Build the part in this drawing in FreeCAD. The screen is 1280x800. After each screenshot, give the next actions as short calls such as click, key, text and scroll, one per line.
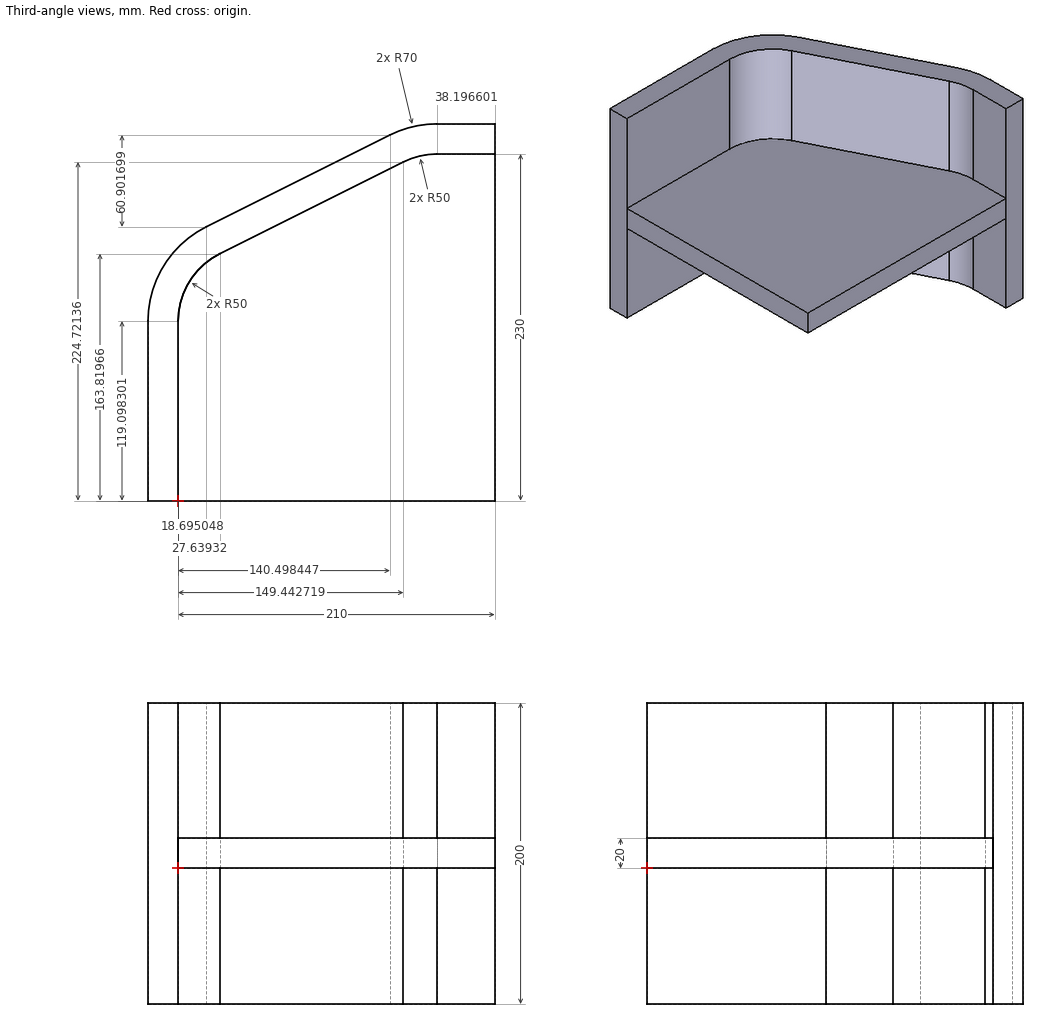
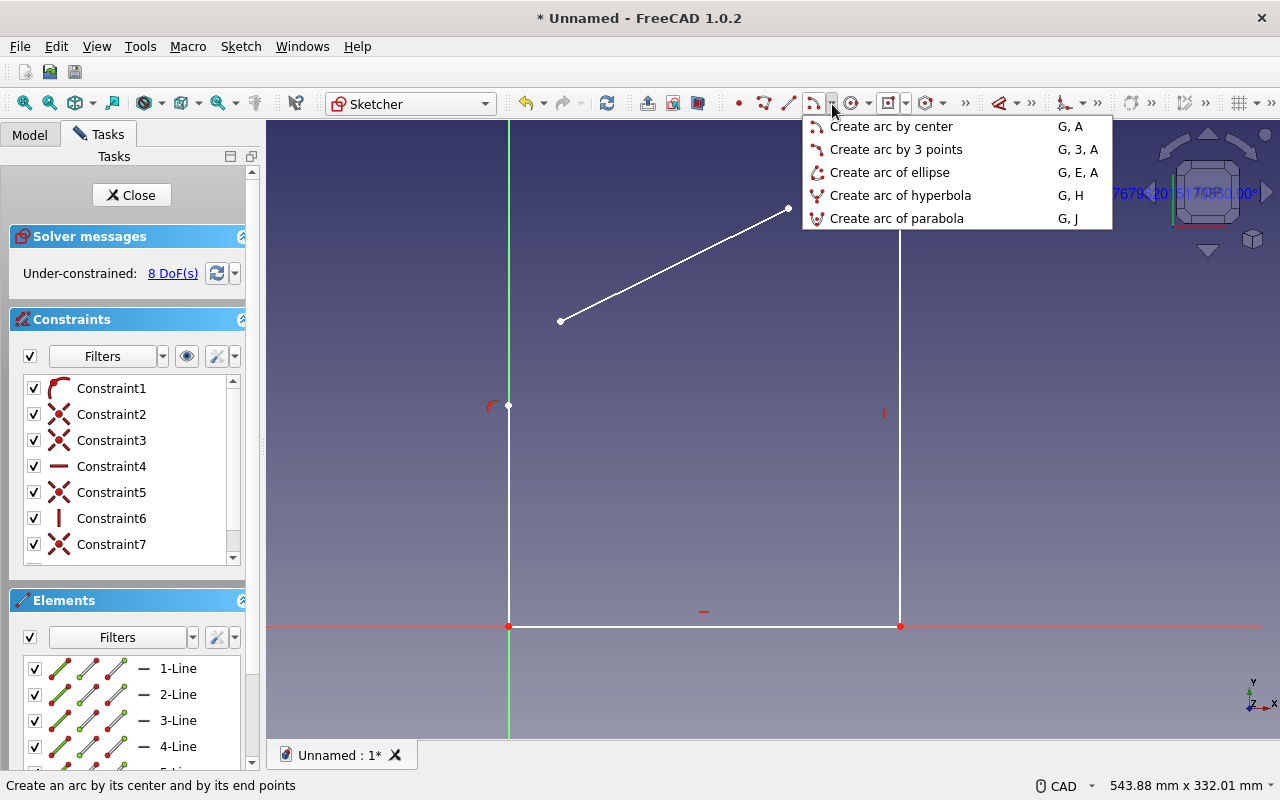
click(958, 150)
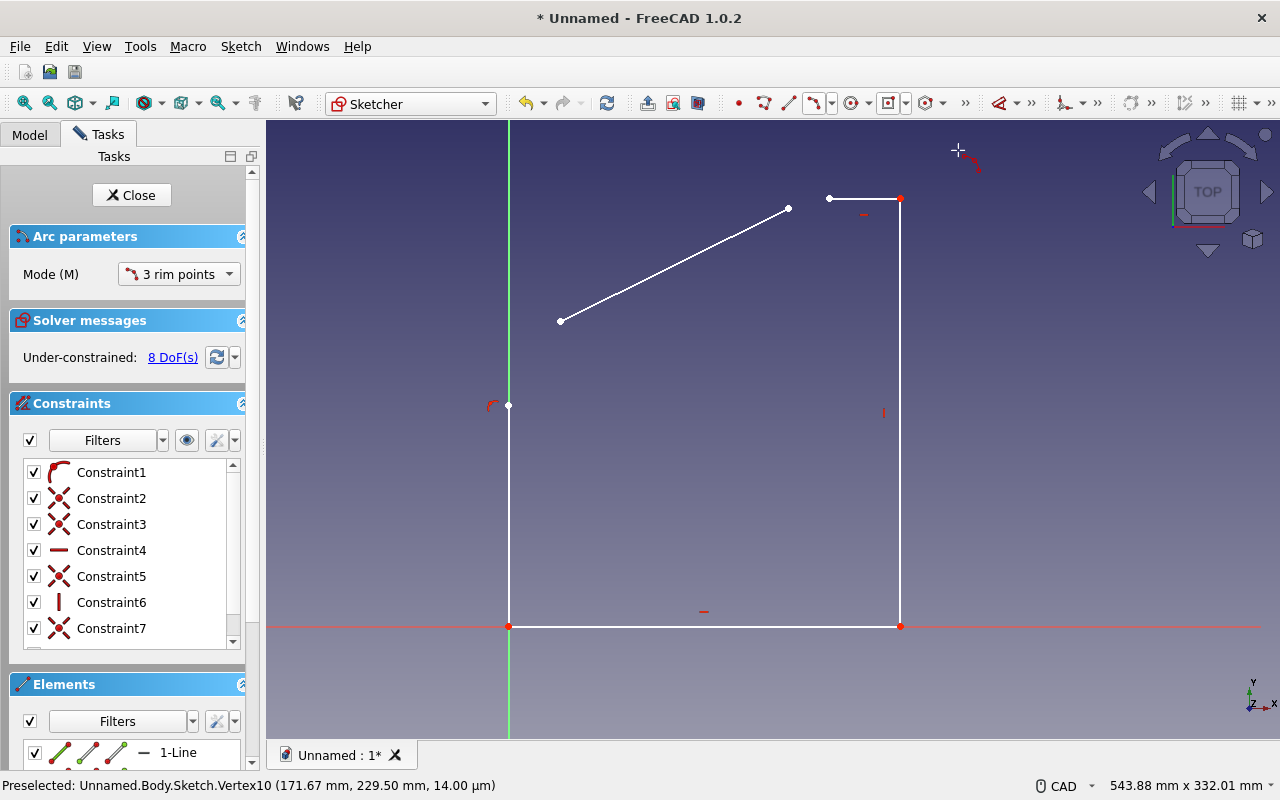
click(560, 322)
click(509, 406)
click(523, 356)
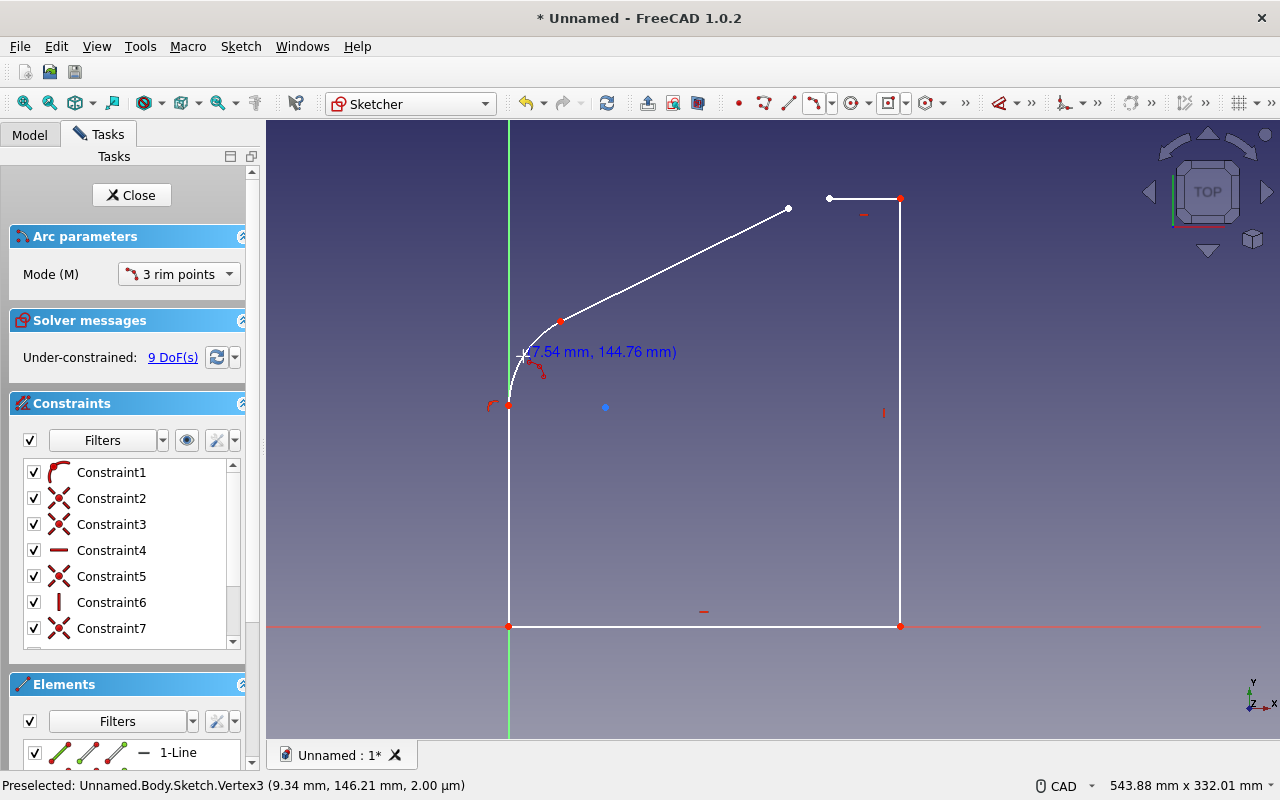
click(829, 199)
click(788, 209)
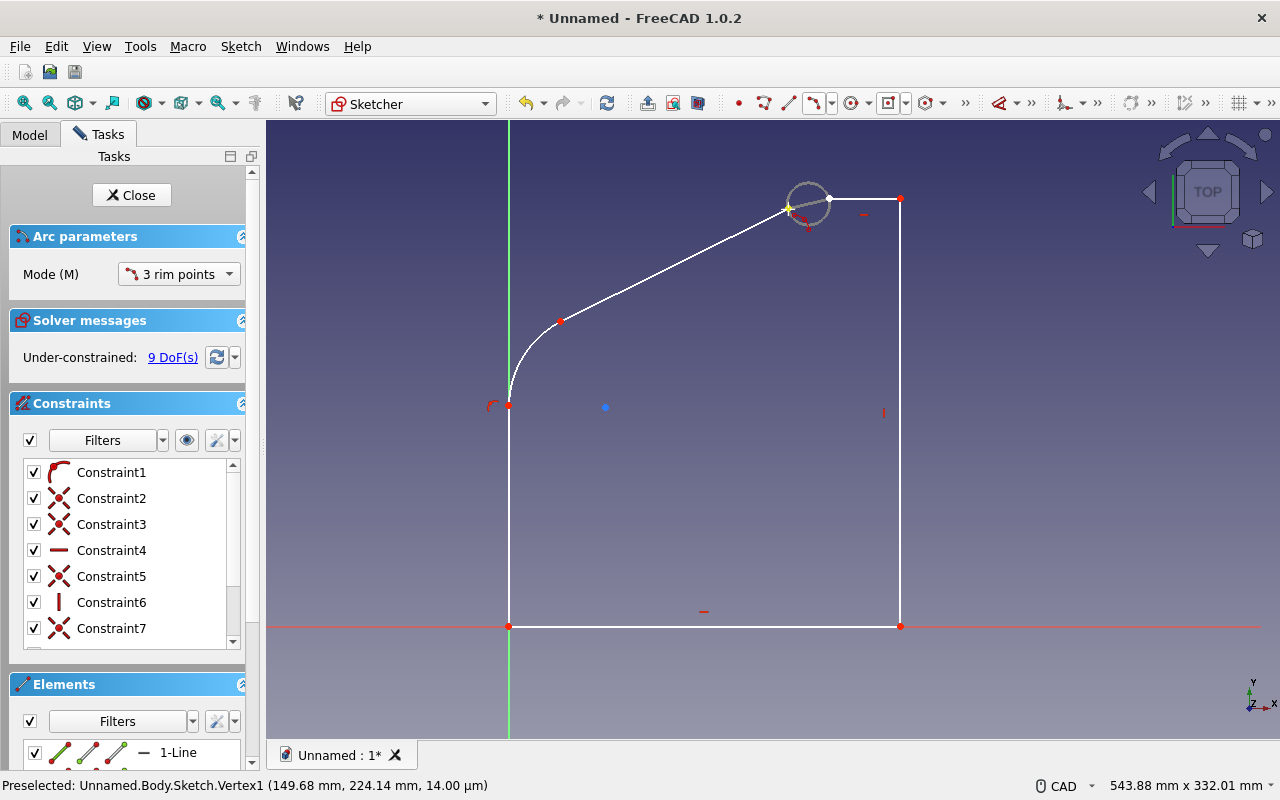
scroll(808, 201, up, 10)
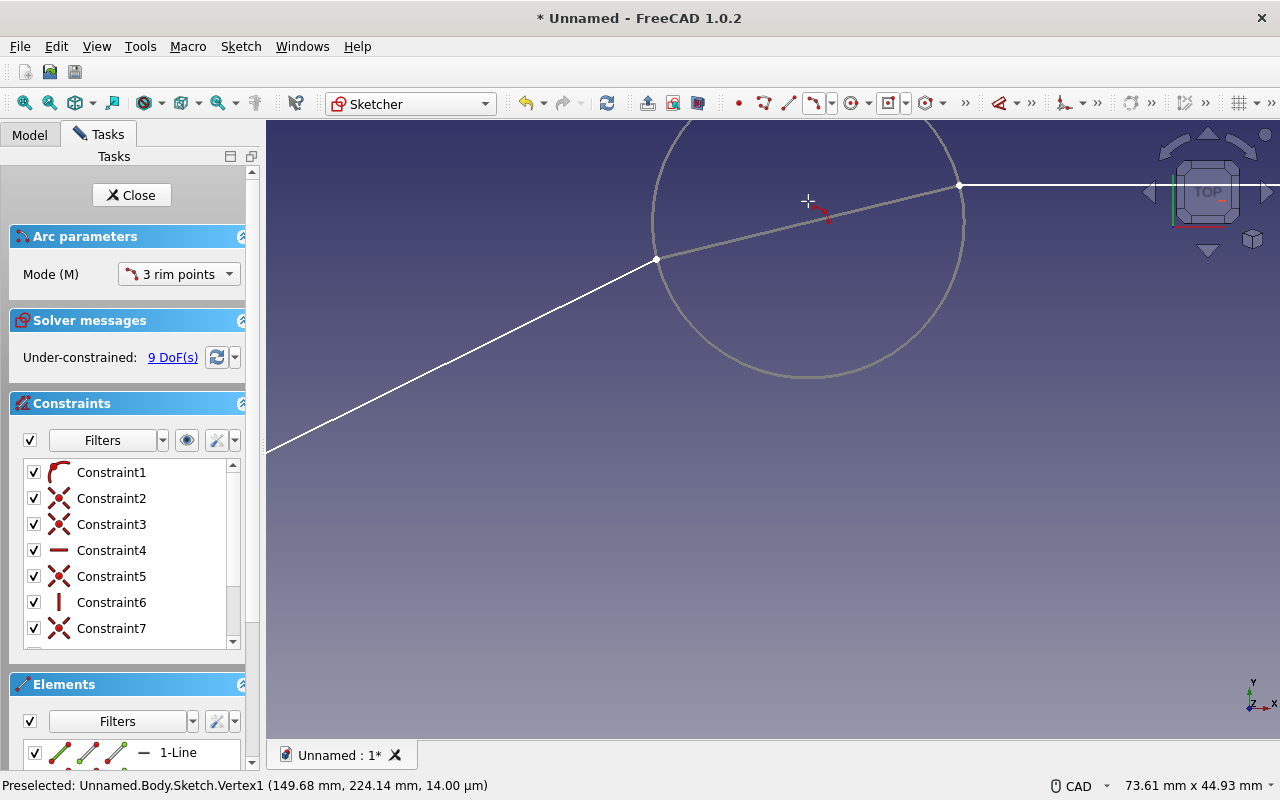
click(803, 197)
key(Escape)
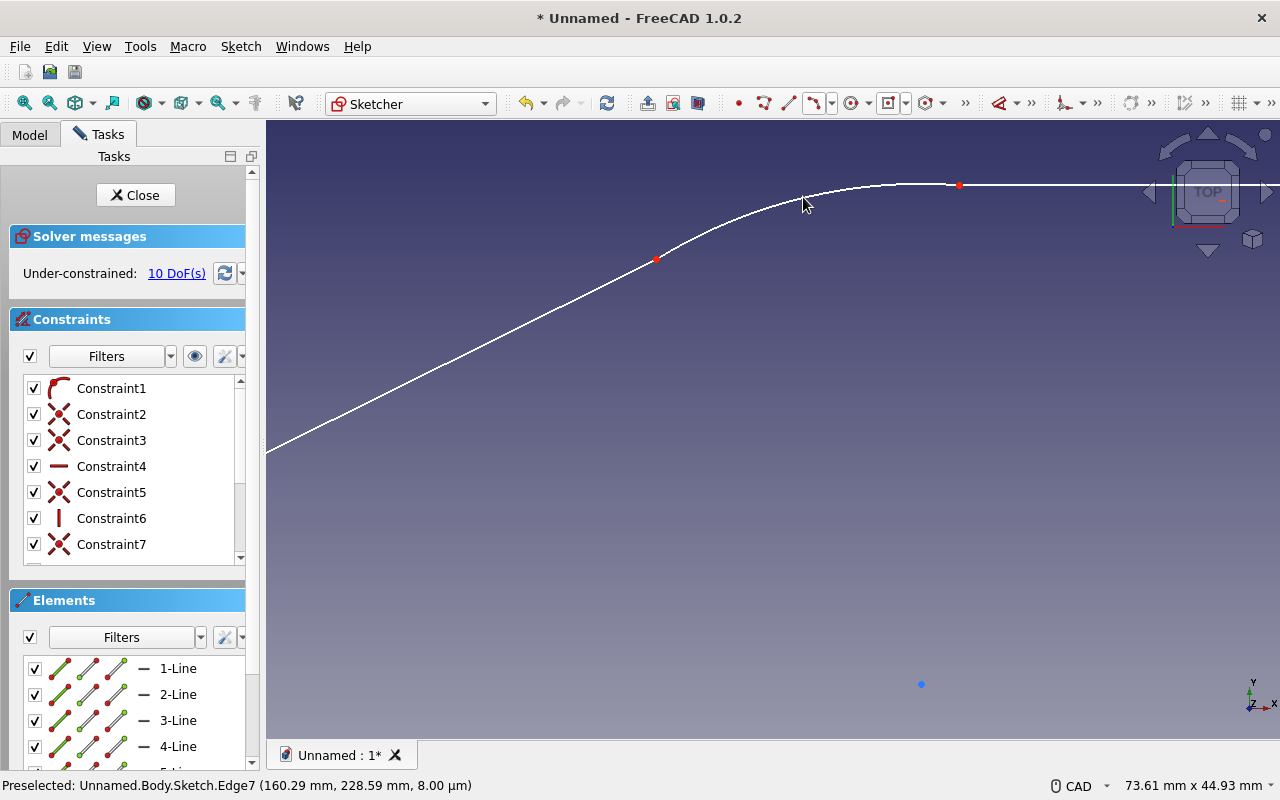
scroll(808, 221, down, 10)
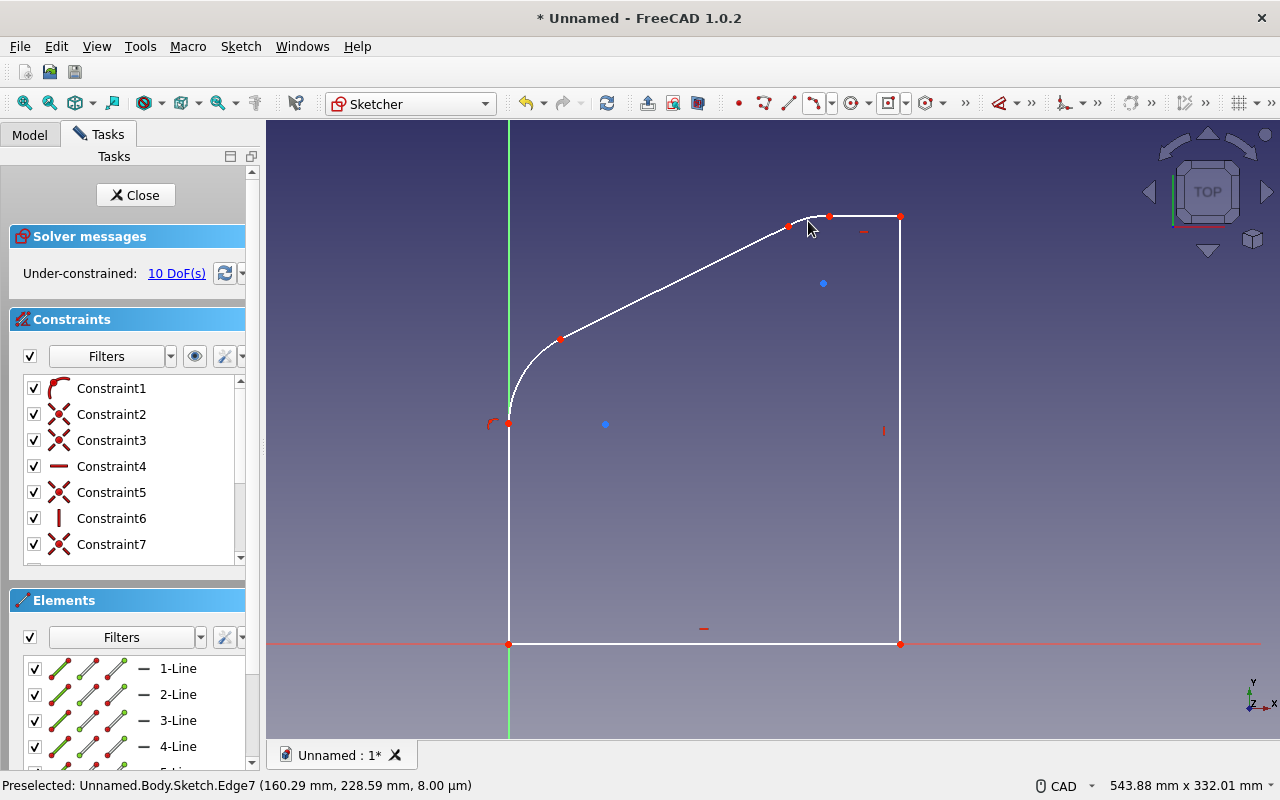
click(535, 358)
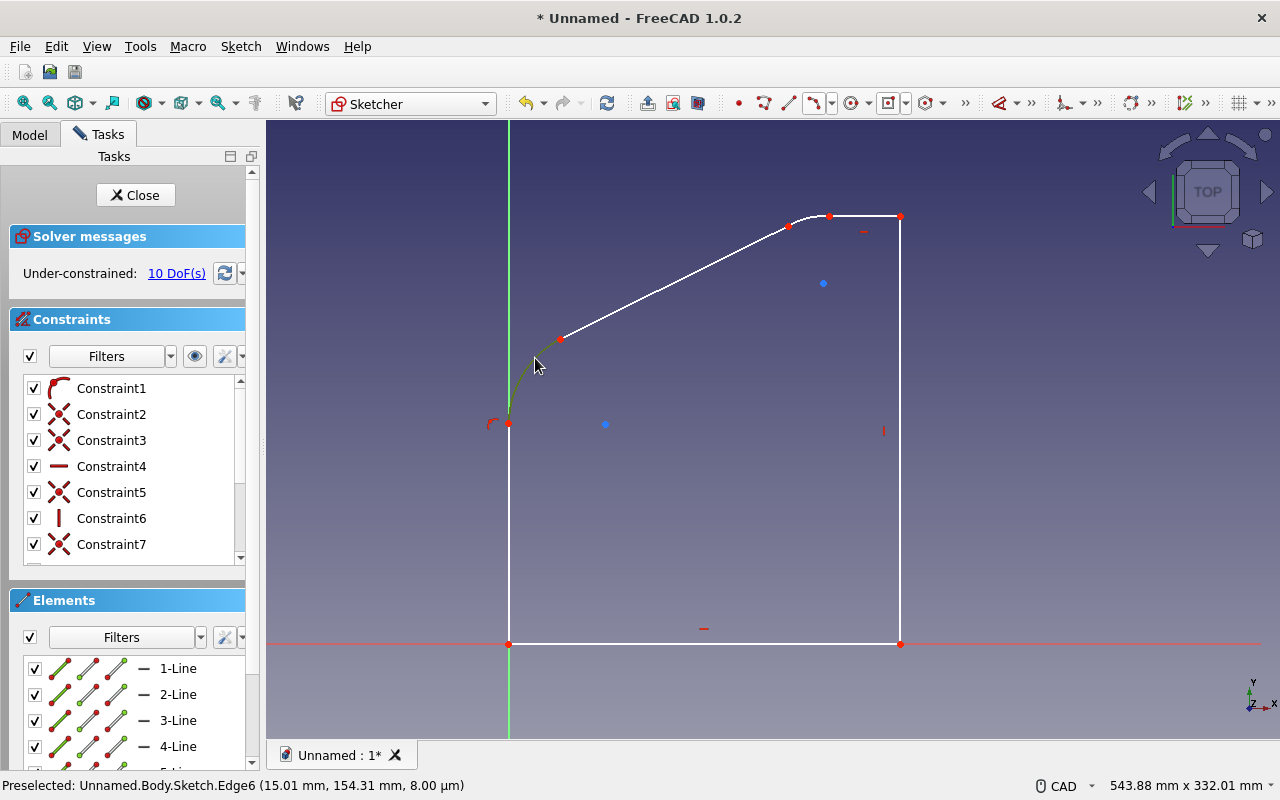
click(816, 217)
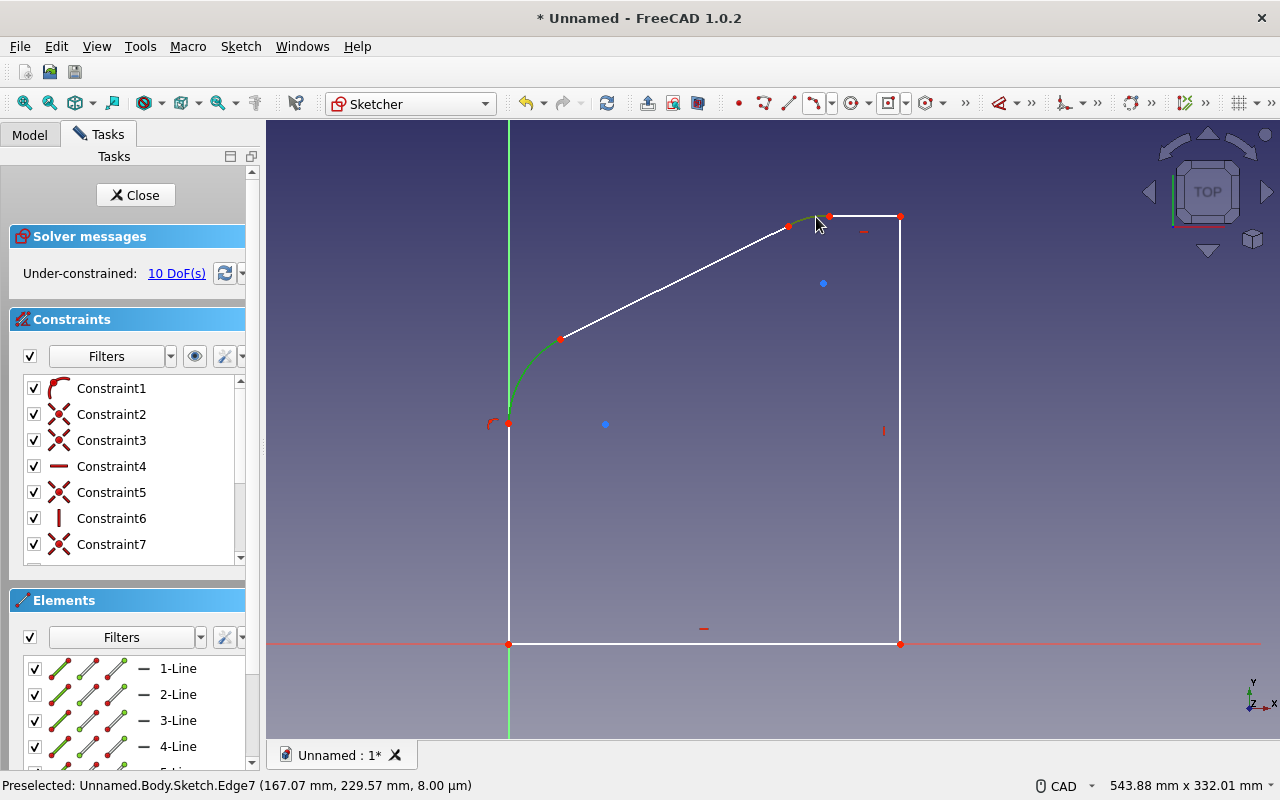
key(e)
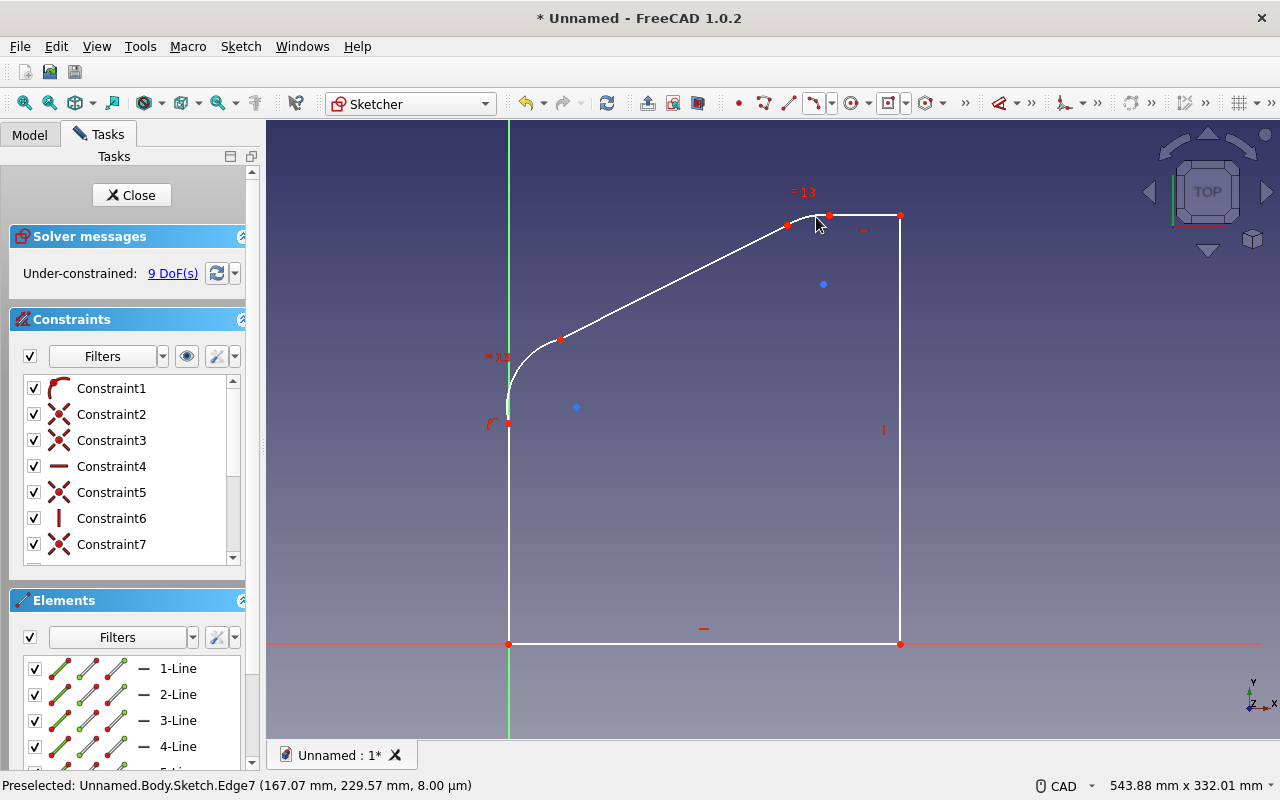
click(998, 104)